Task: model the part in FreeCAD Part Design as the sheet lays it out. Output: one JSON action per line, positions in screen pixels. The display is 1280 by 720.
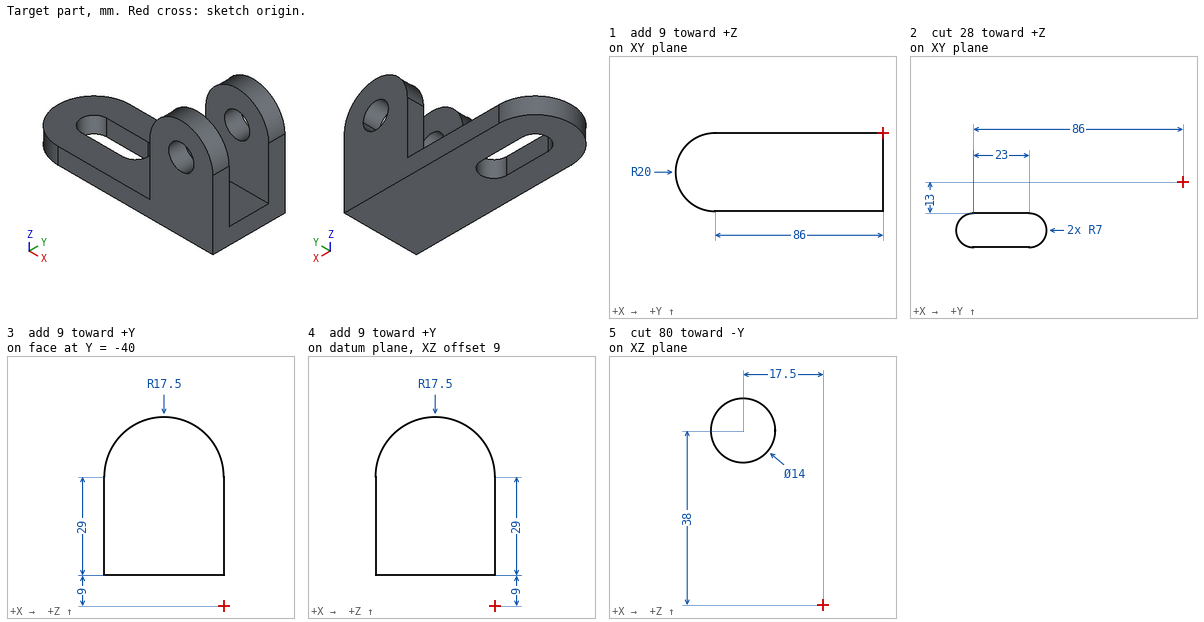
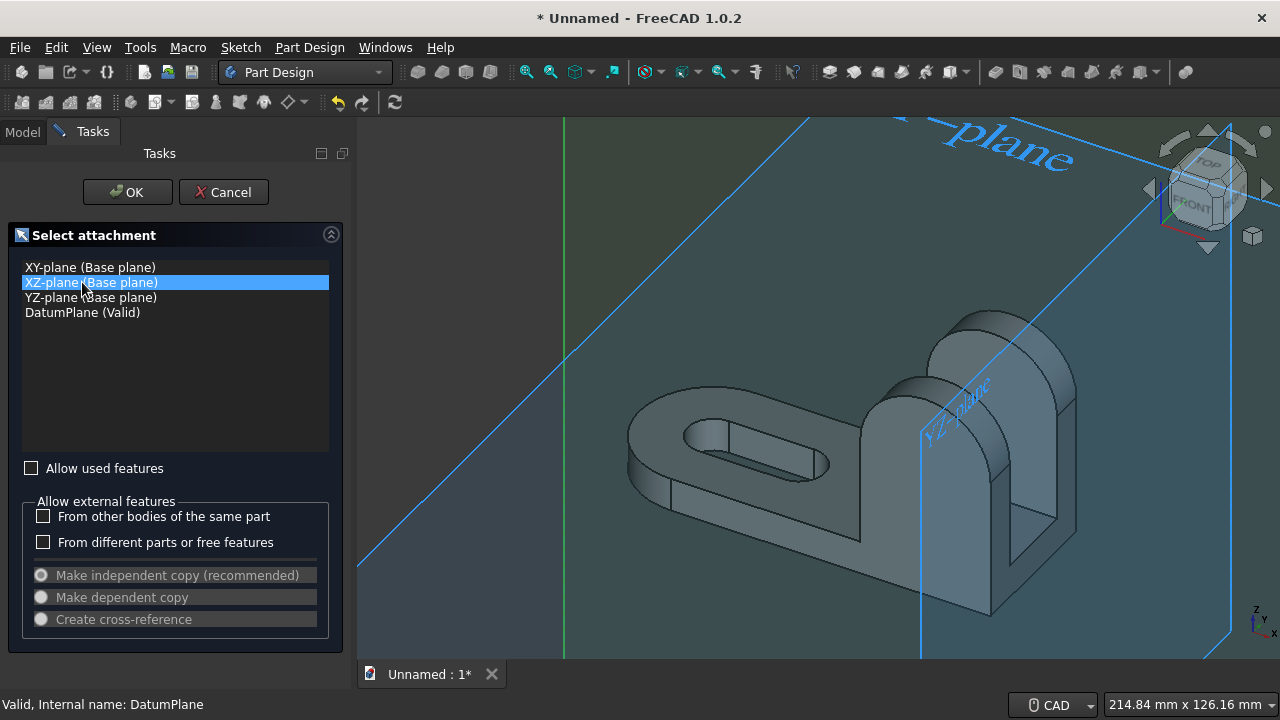
{"action": "left_click", "coordinate": [128, 192]}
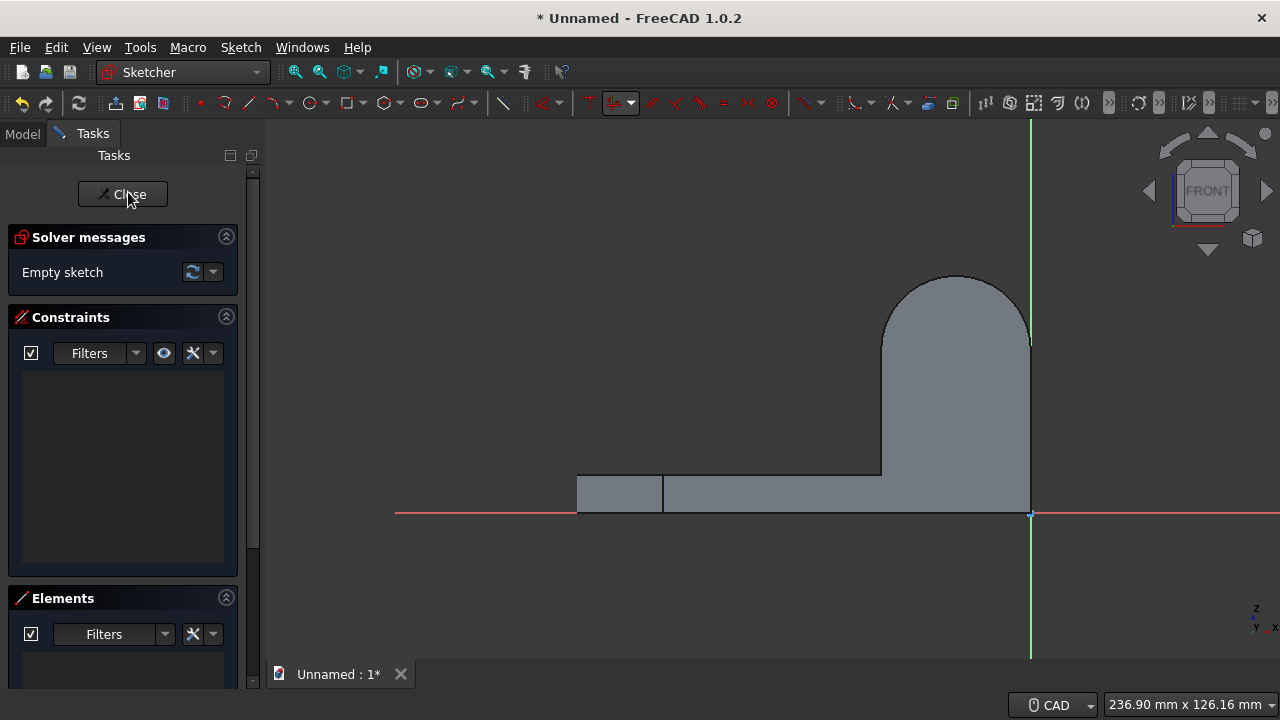
{"action": "left_click", "coordinate": [164, 104]}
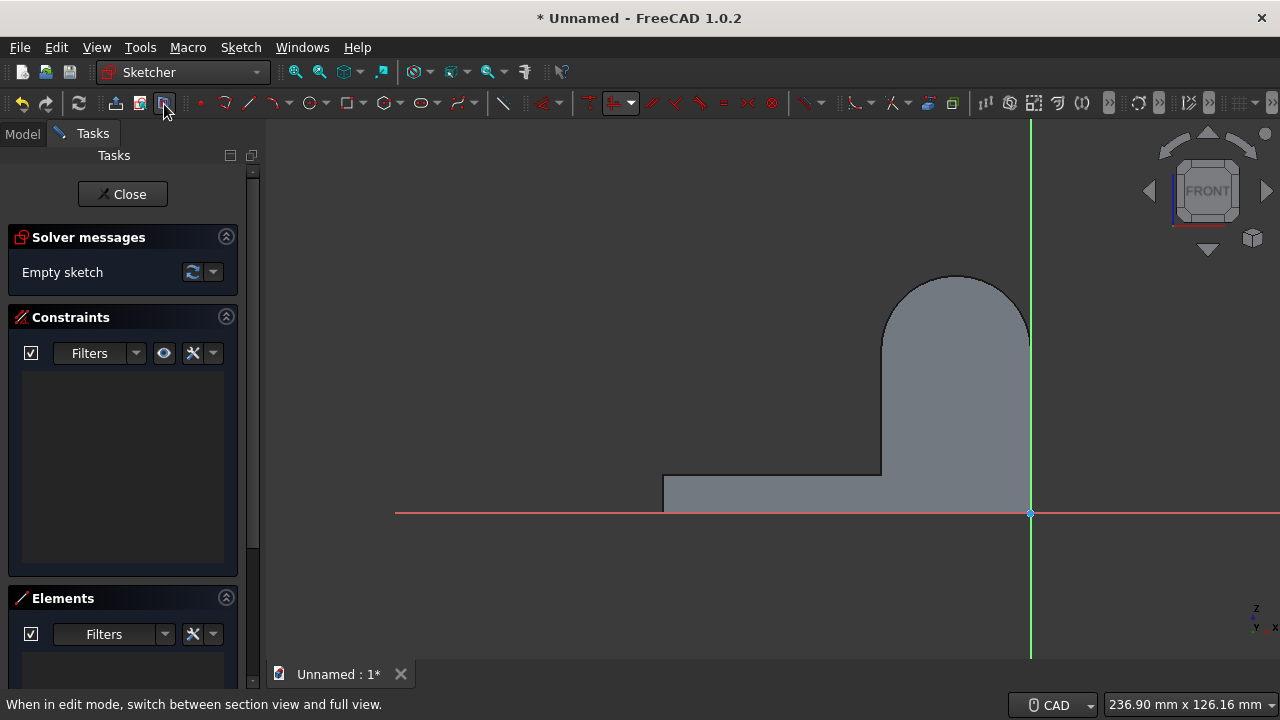
{"action": "scroll", "coordinate": [1006, 343], "scroll_direction": "up", "scroll_amount": 9}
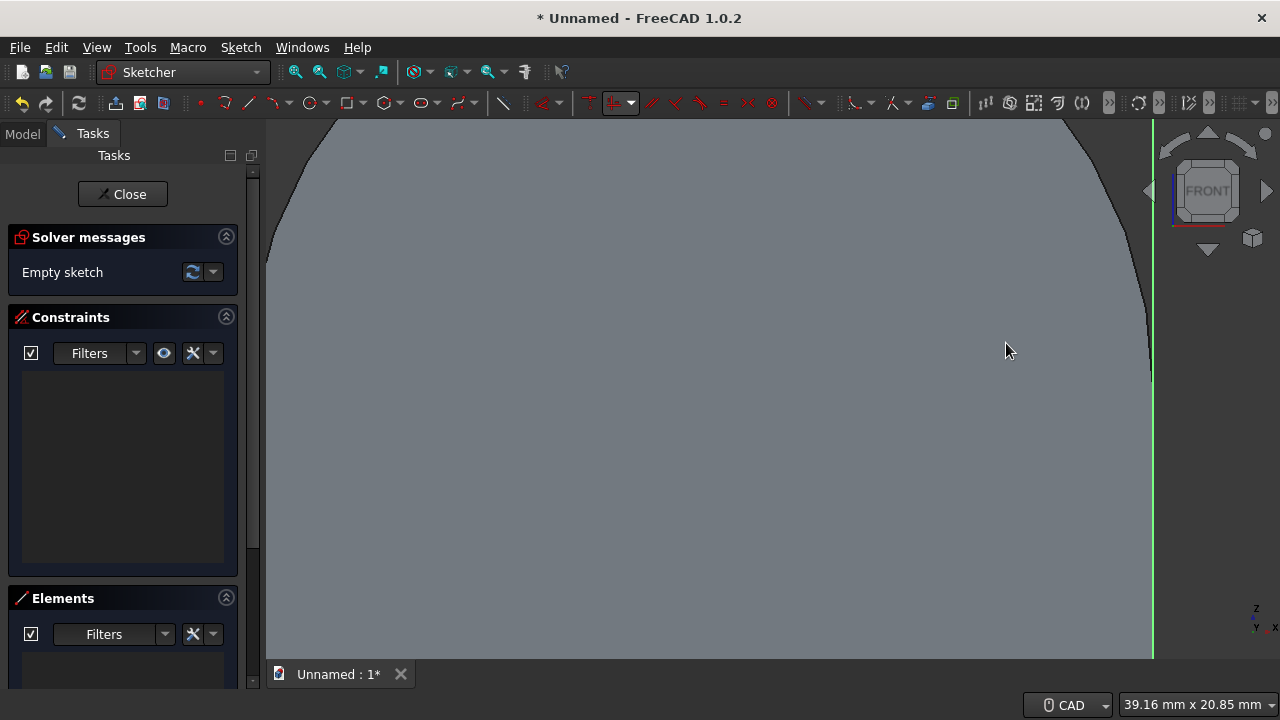
{"action": "left_click", "coordinate": [310, 104]}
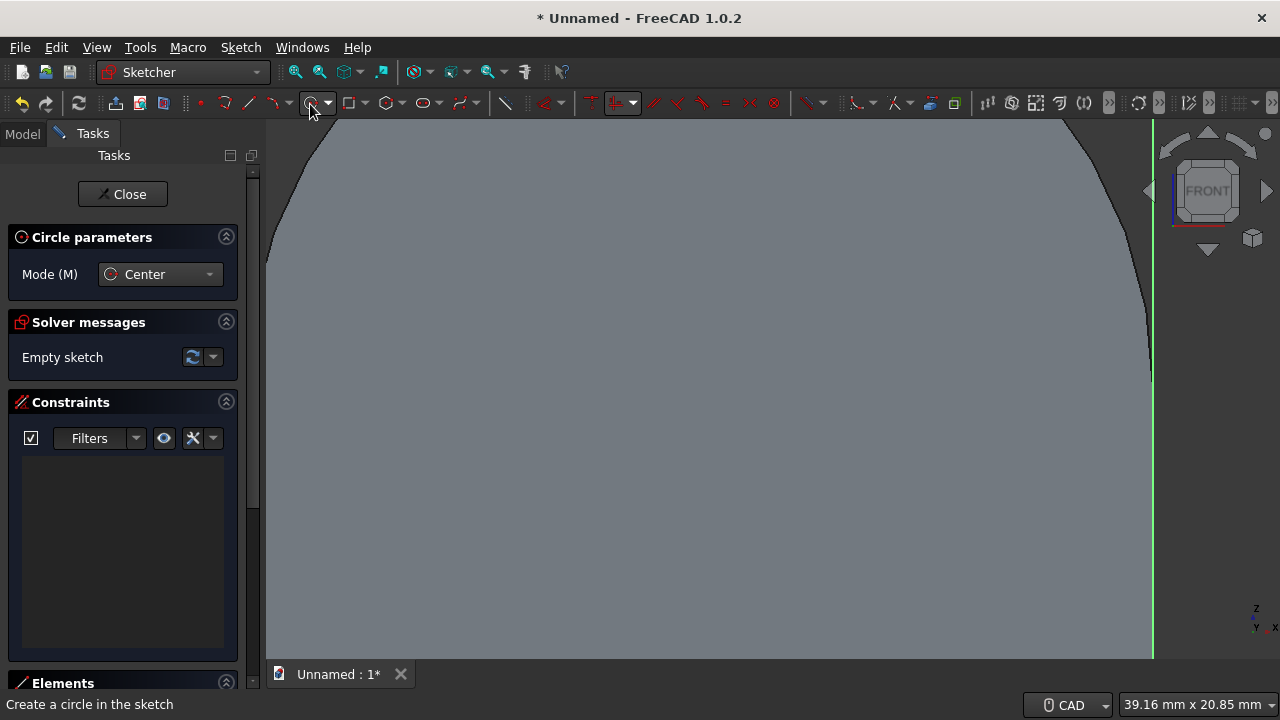
{"action": "left_click", "coordinate": [700, 388]}
{"action": "mouse_move", "coordinate": [828, 259]}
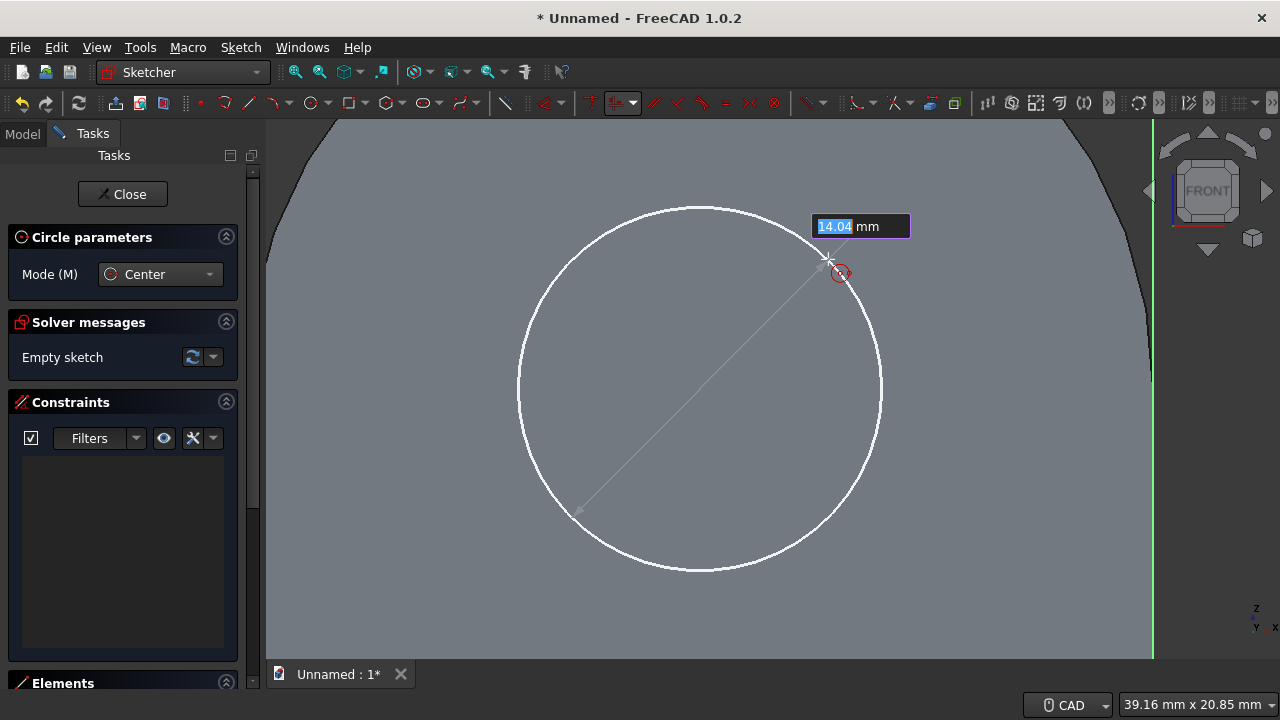
{"action": "type", "text": "14"}
{"action": "key", "text": "Return"}
{"action": "key", "text": "Escape"}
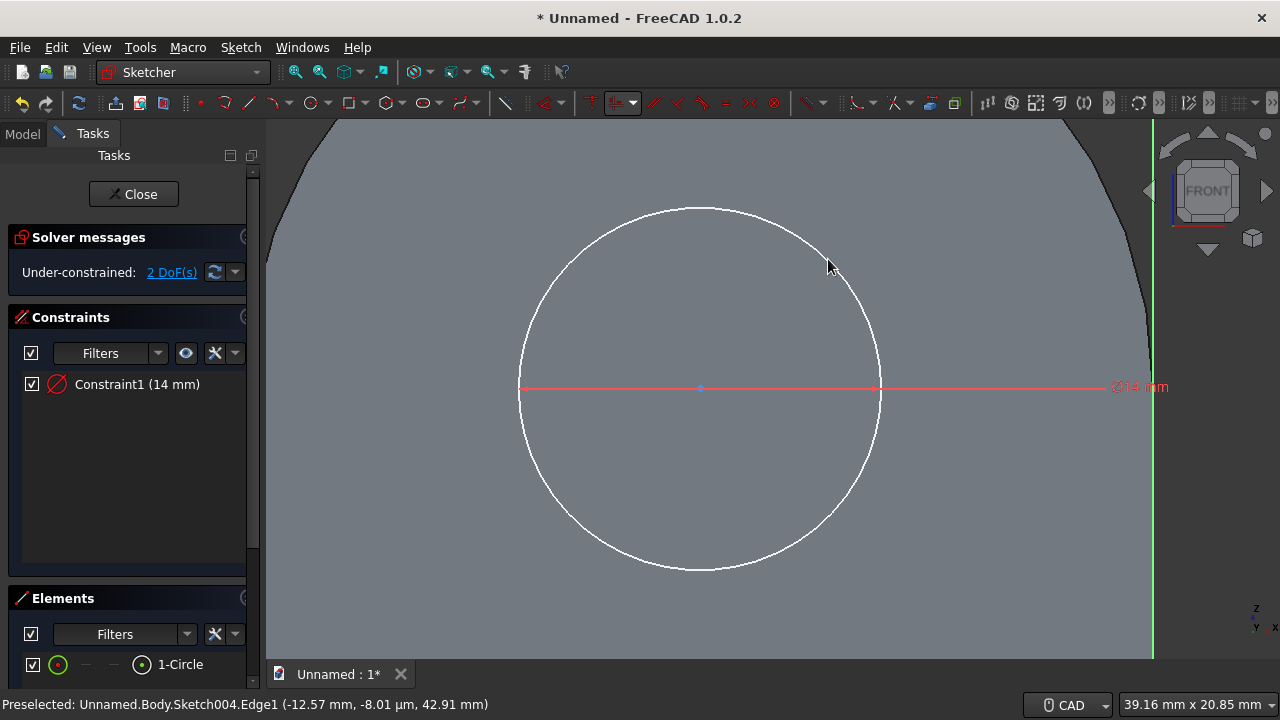
{"action": "left_click", "coordinate": [544, 104]}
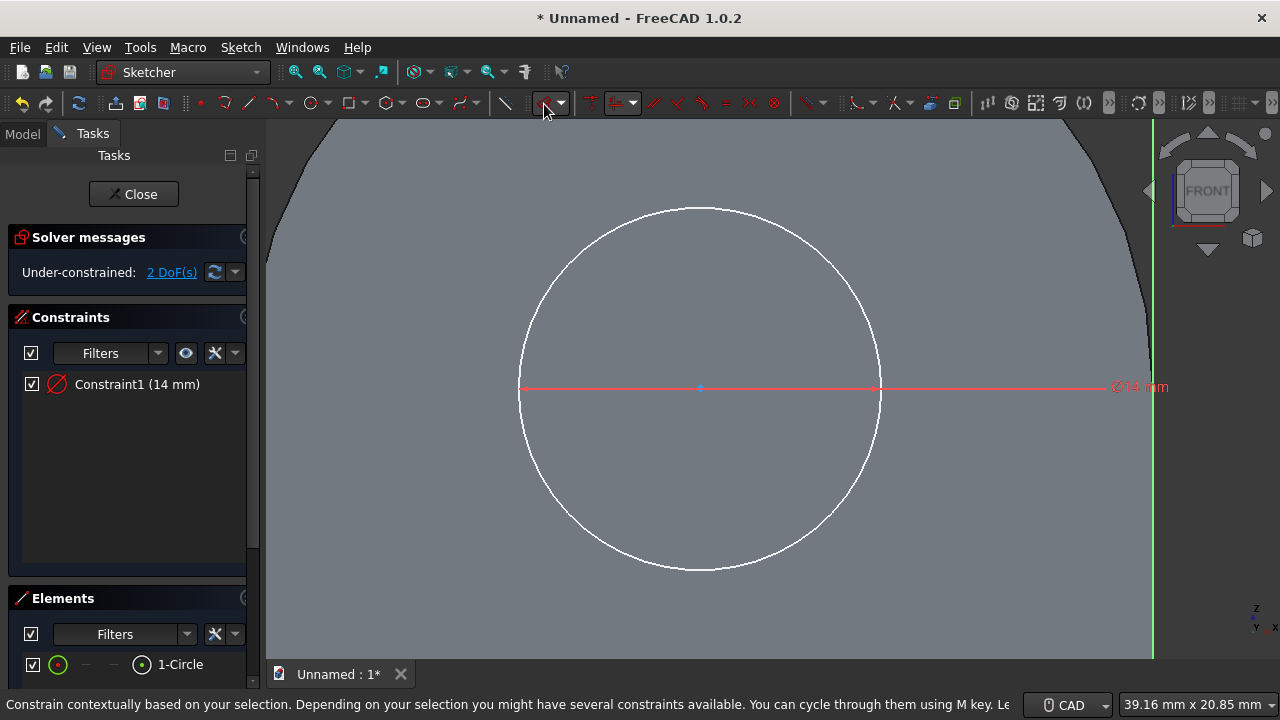
{"action": "left_click", "coordinate": [700, 389]}
{"action": "left_click", "coordinate": [666, 510]}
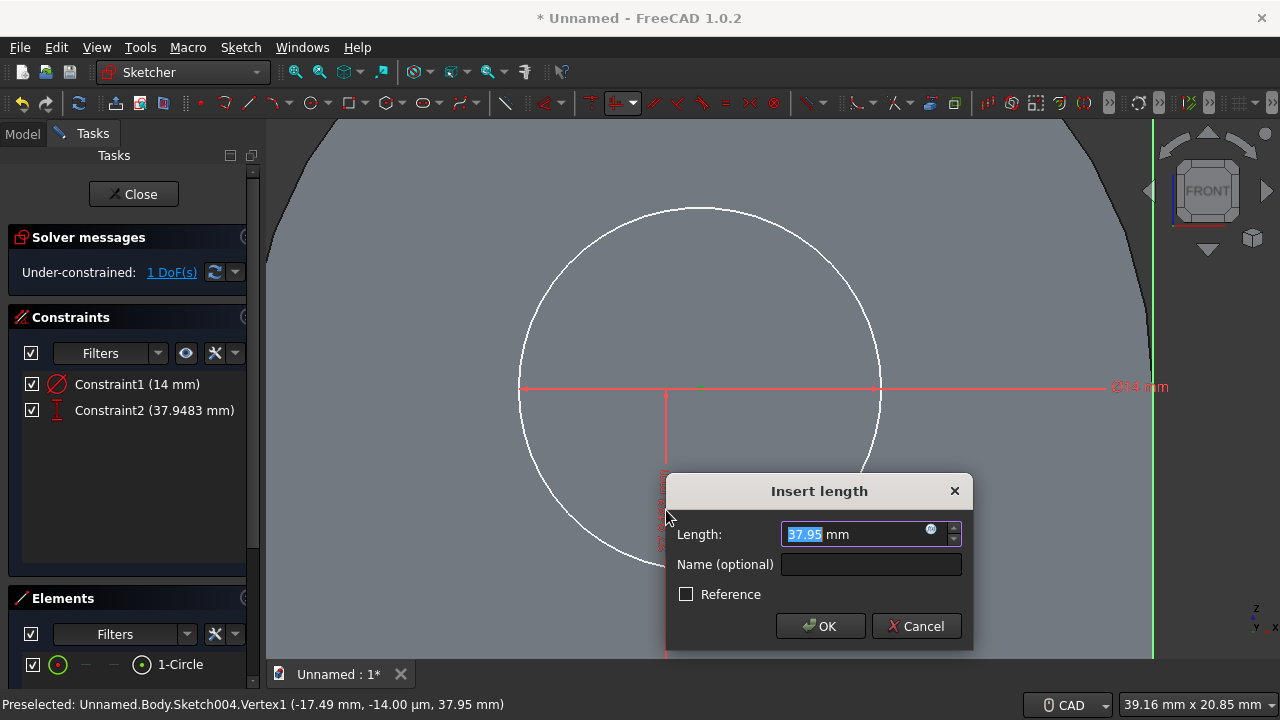
{"action": "type", "text": "38"}
{"action": "key", "text": "Return"}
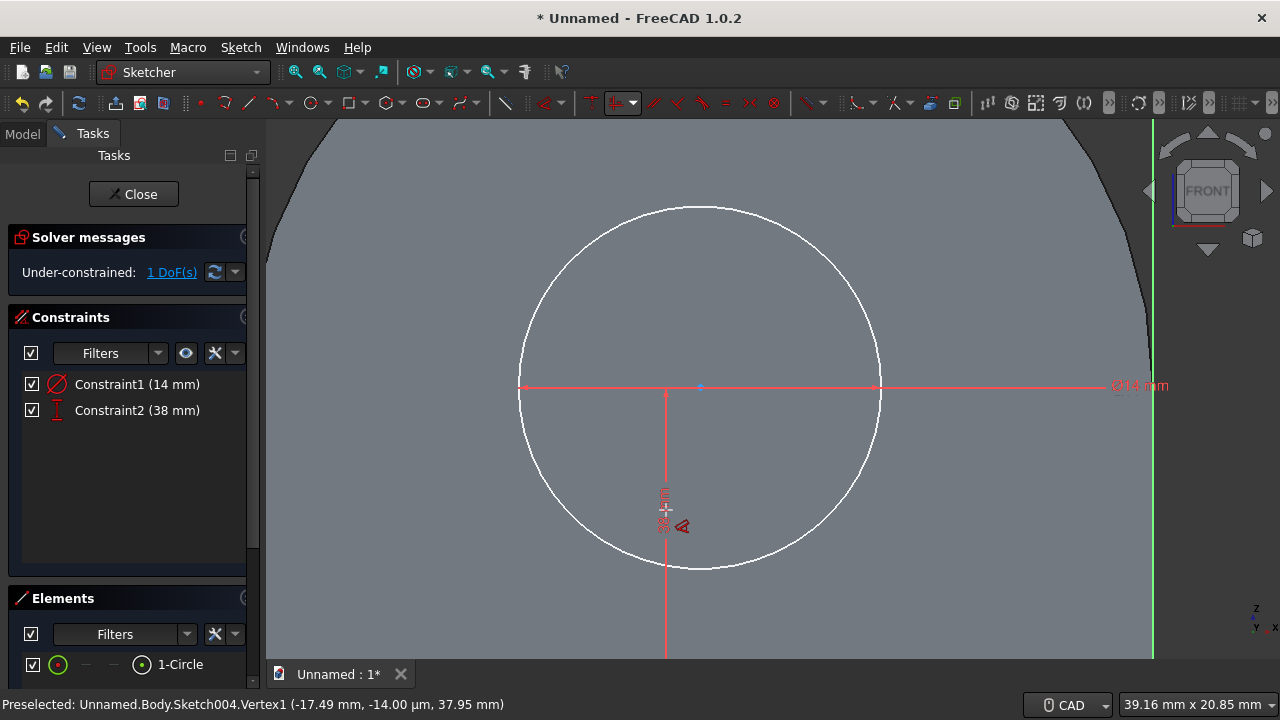
{"action": "left_click", "coordinate": [700, 388]}
{"action": "left_click", "coordinate": [907, 354]}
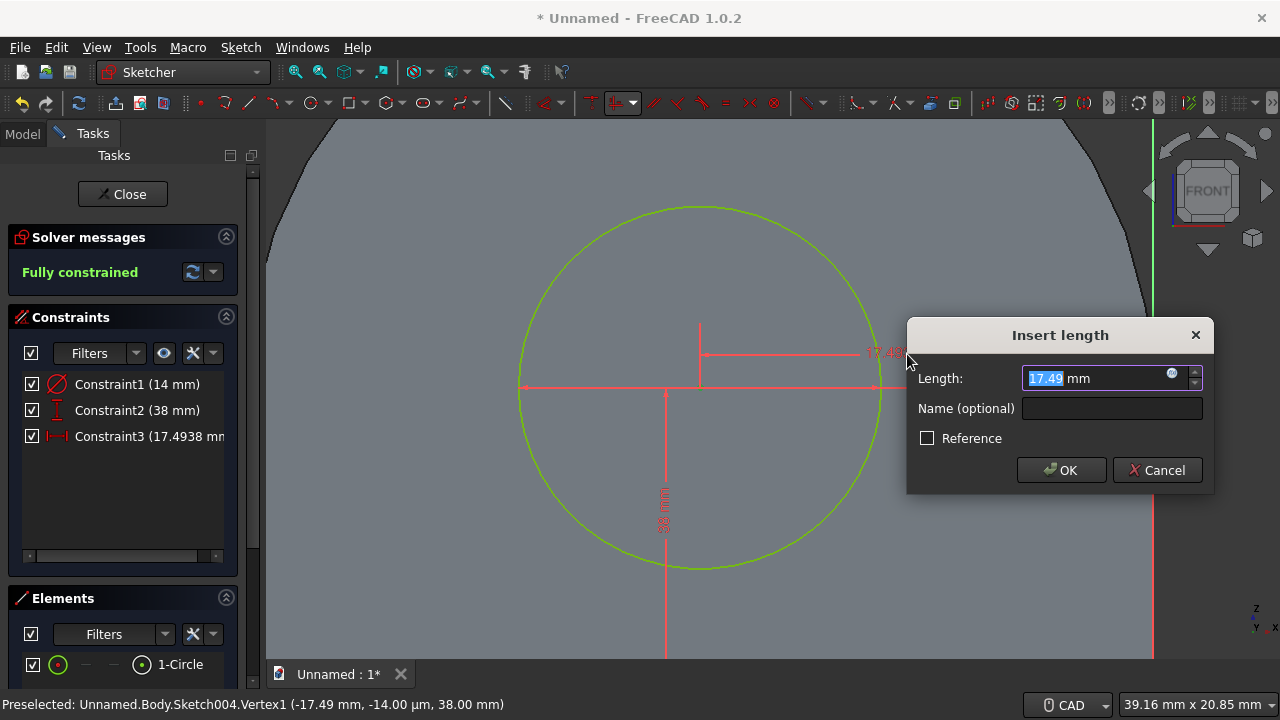
{"action": "type", "text": "17.5"}
{"action": "key", "text": "Return"}
{"action": "key", "text": "Escape"}